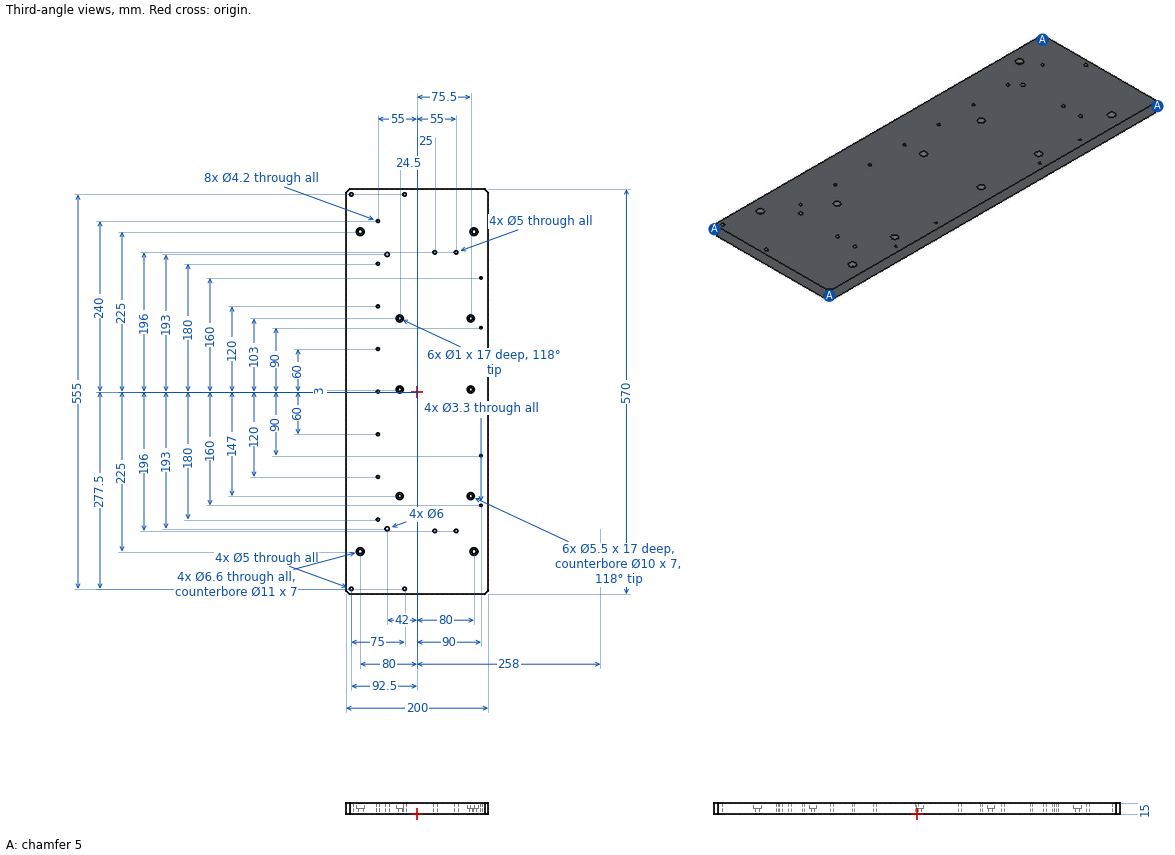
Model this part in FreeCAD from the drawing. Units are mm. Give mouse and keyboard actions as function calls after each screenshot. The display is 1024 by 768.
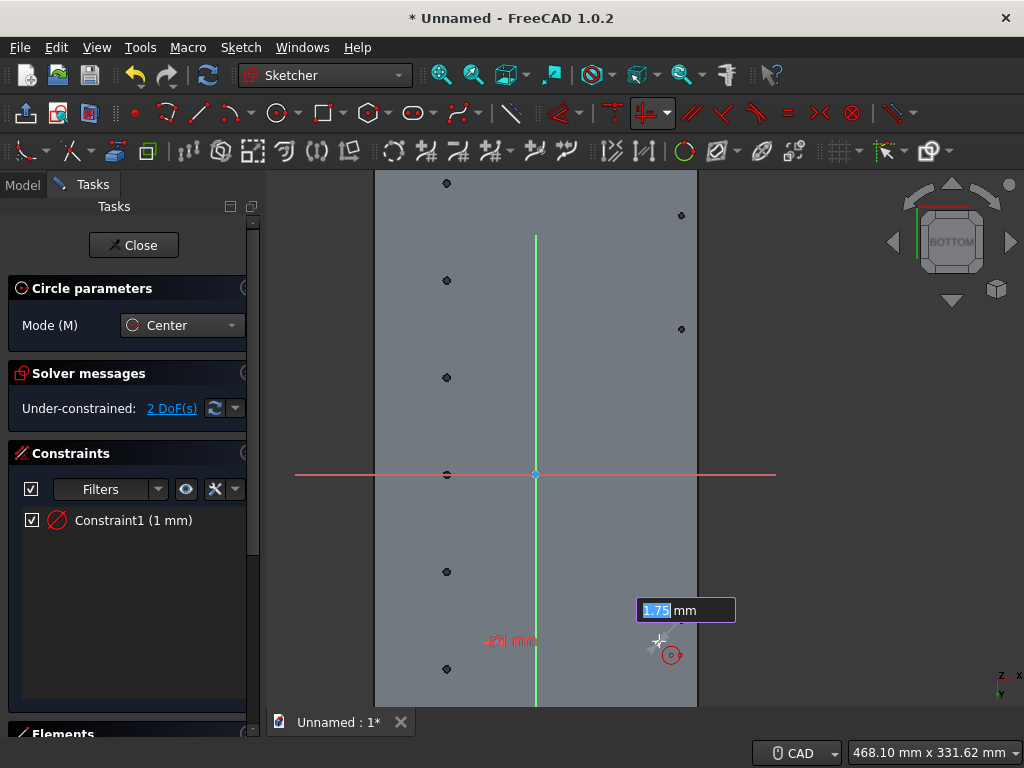
text(1)
key(Return)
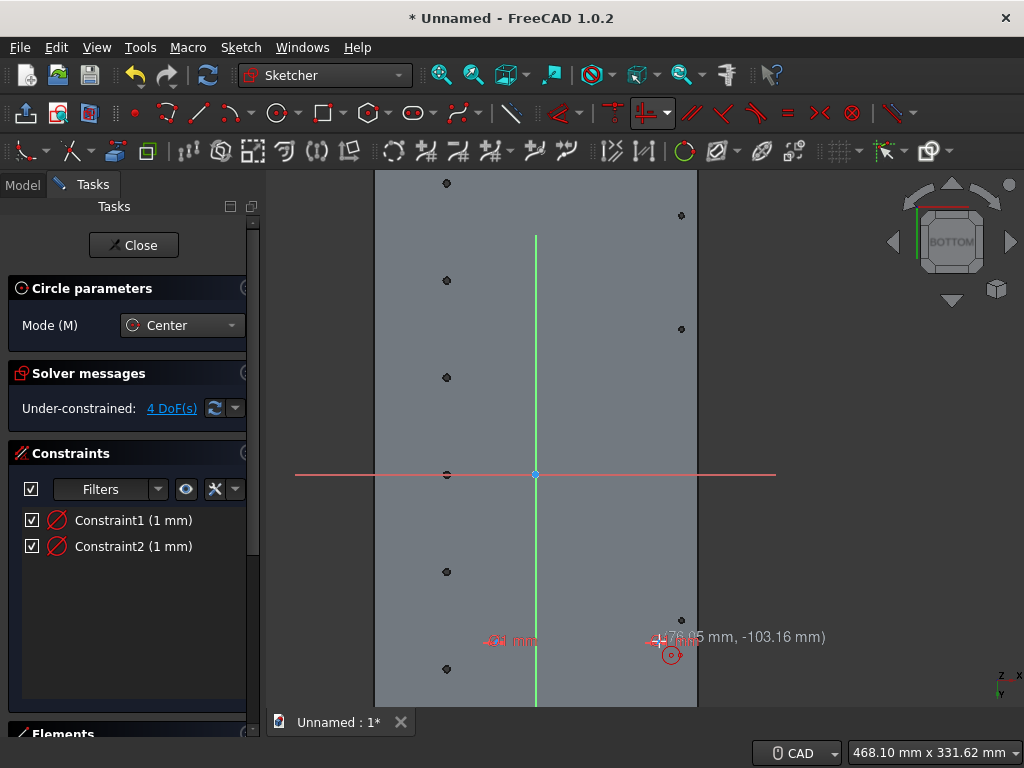
scroll(496, 237, up, 17)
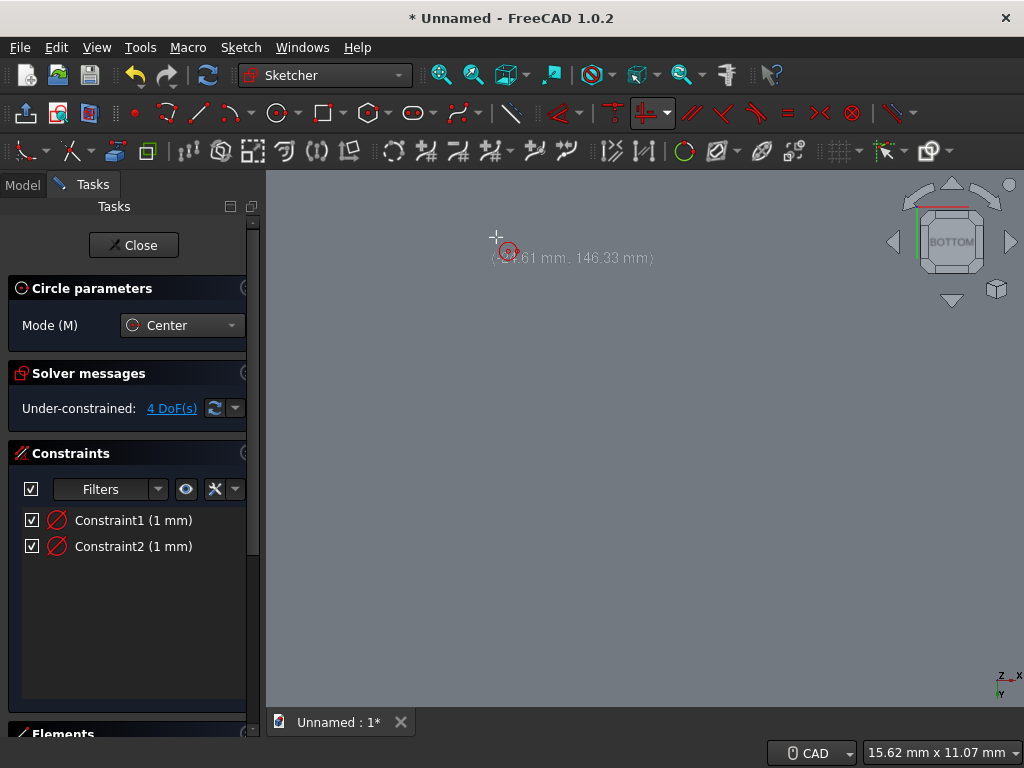
scroll(496, 236, down, 17)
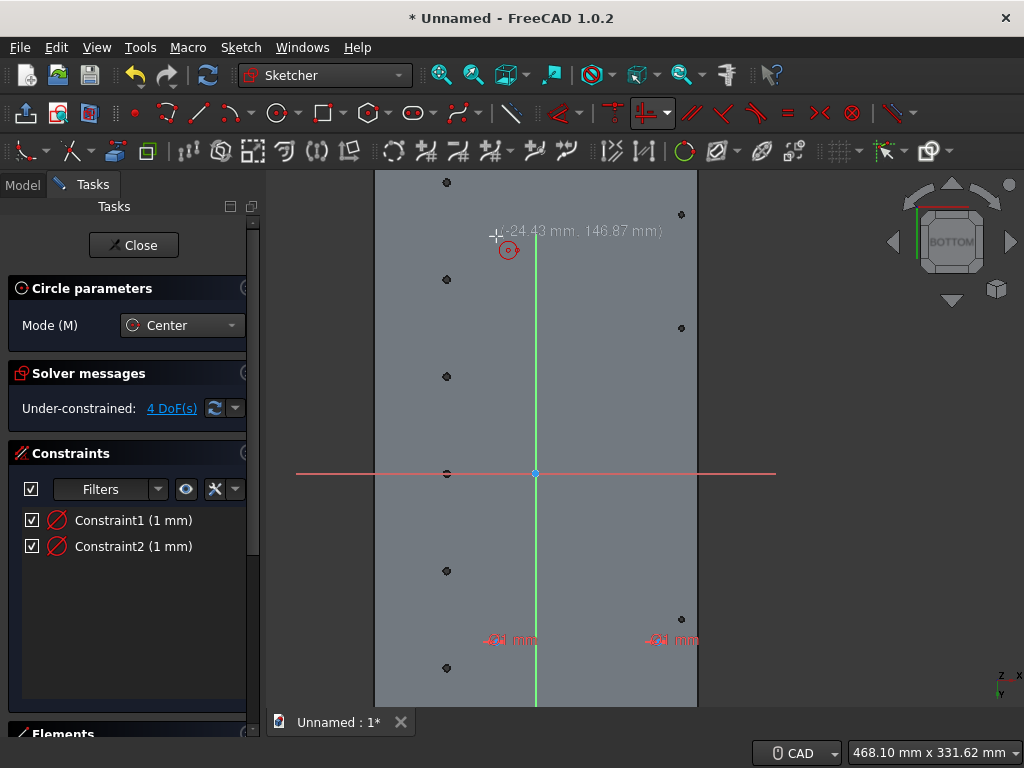
click(496, 236)
move(497, 235)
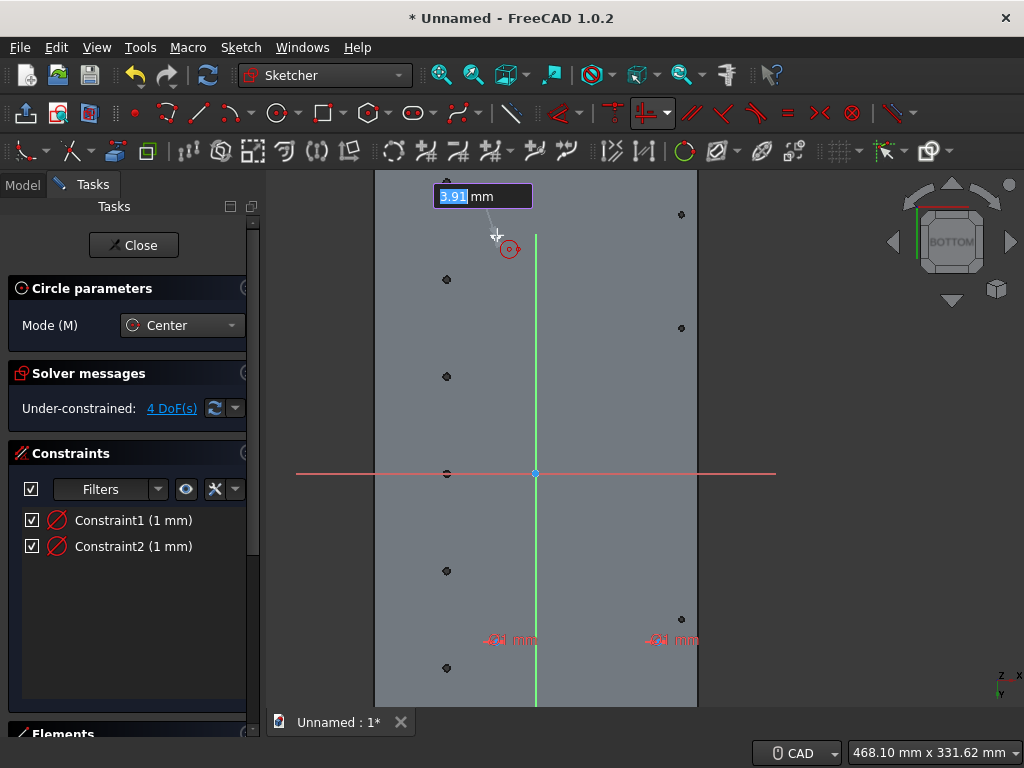
text(1)
key(Return)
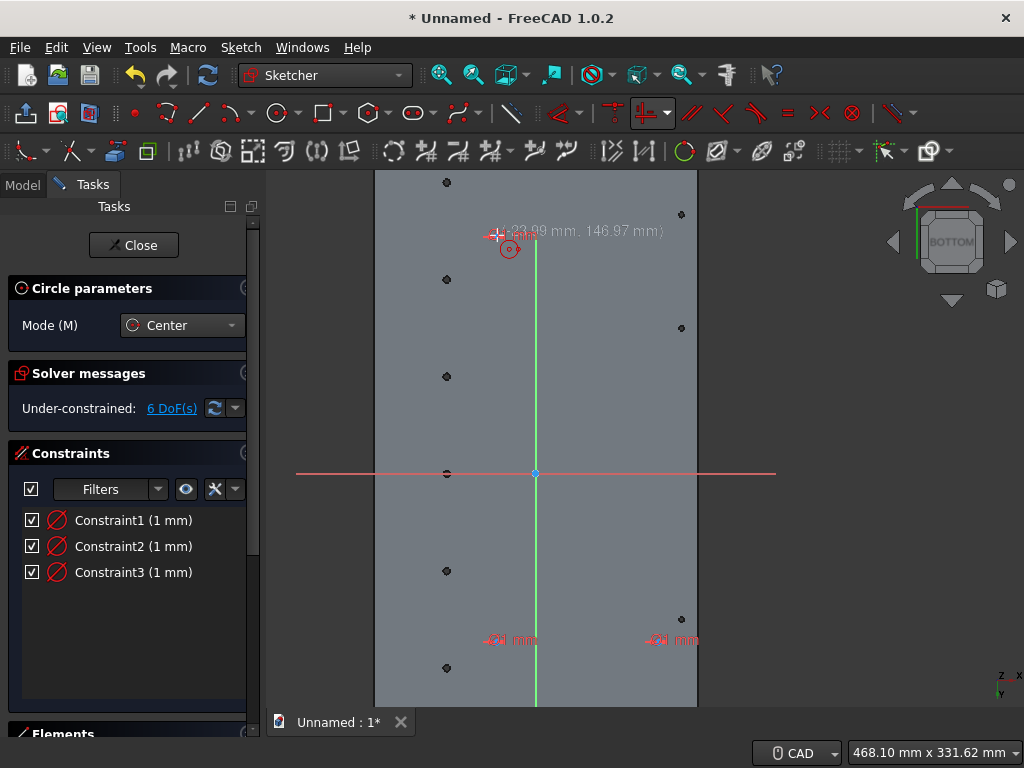
scroll(658, 236, up, 17)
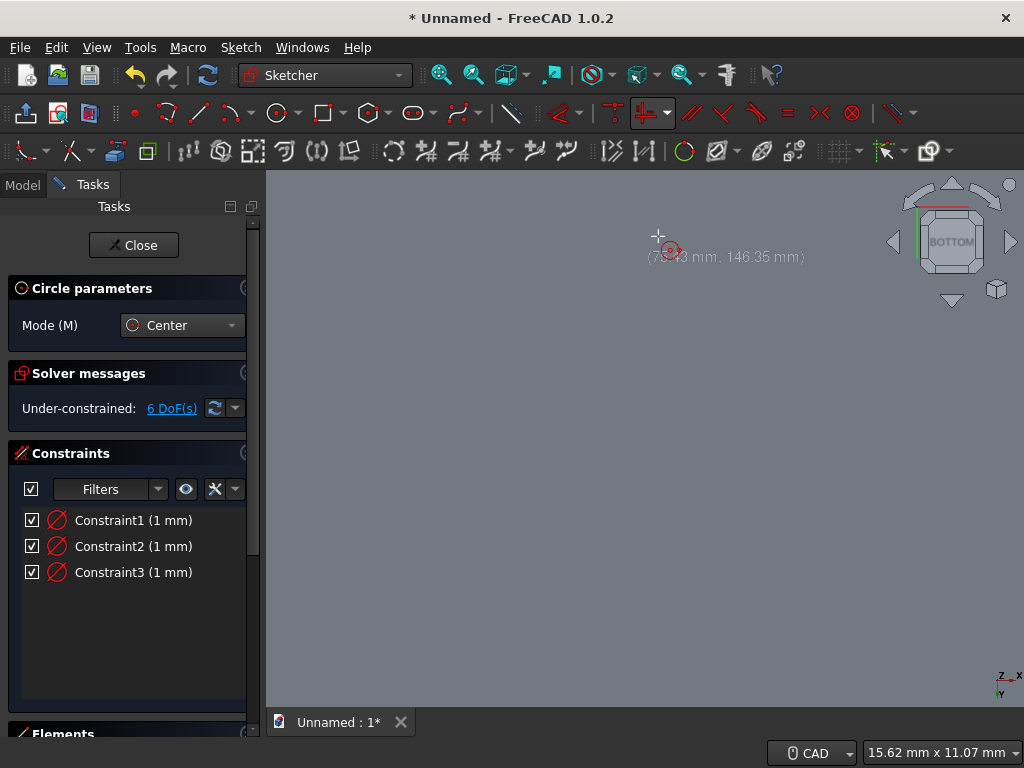
scroll(658, 236, down, 17)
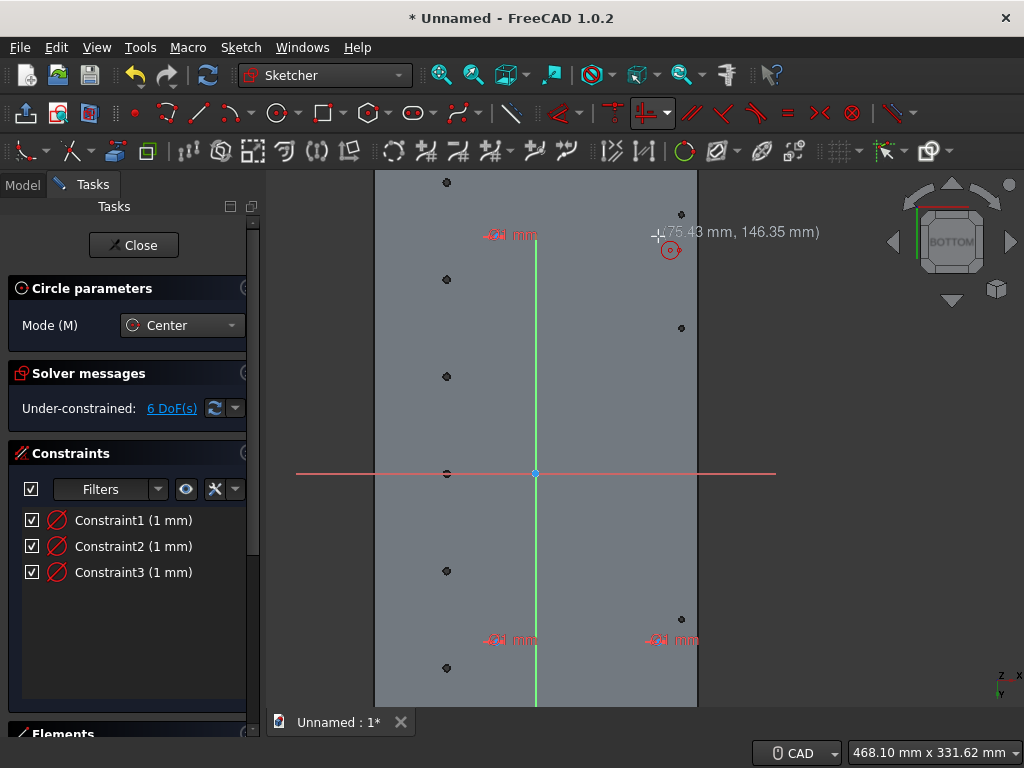
click(658, 236)
move(659, 235)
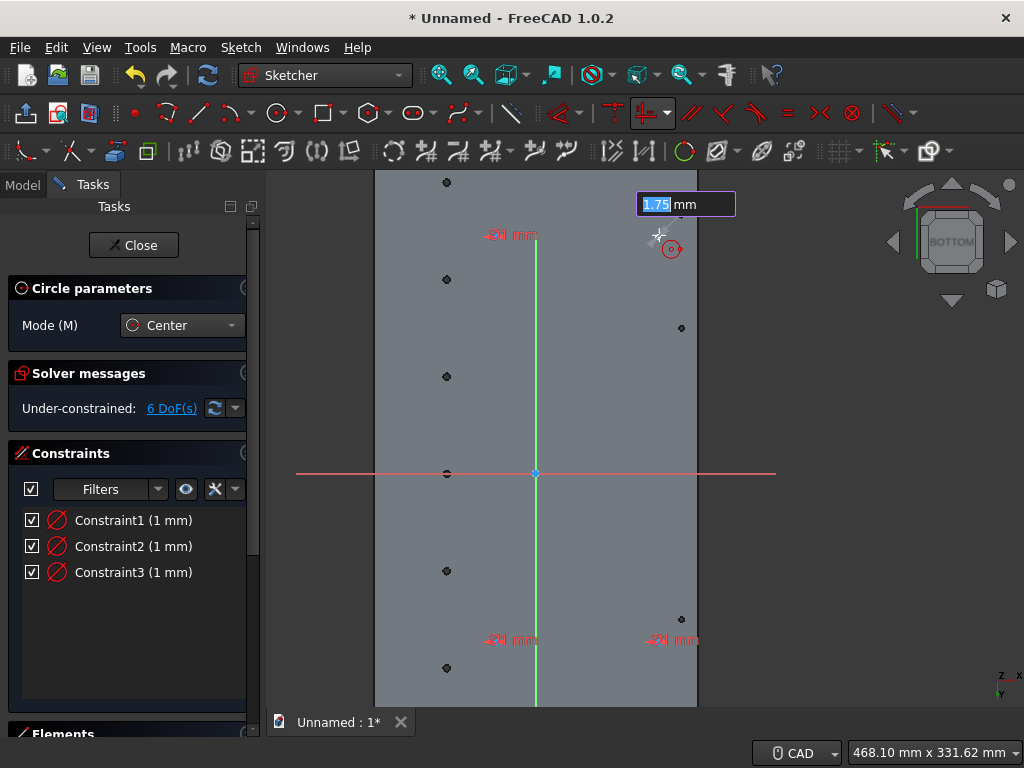
text(1)
key(Return)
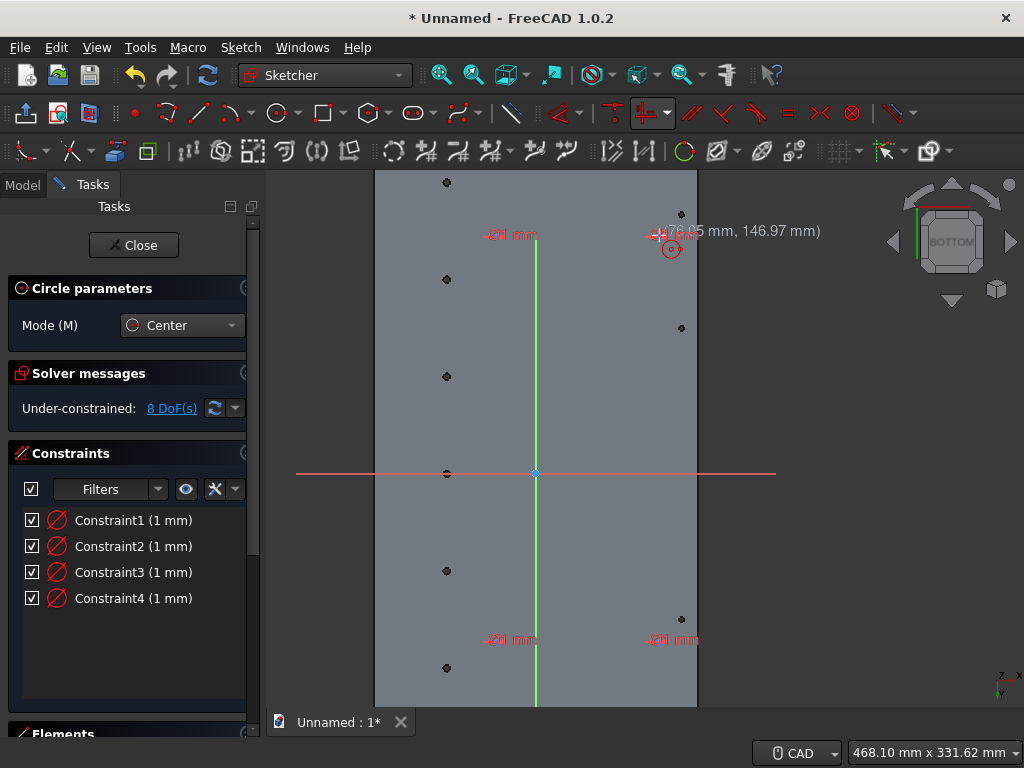
scroll(496, 479, up, 17)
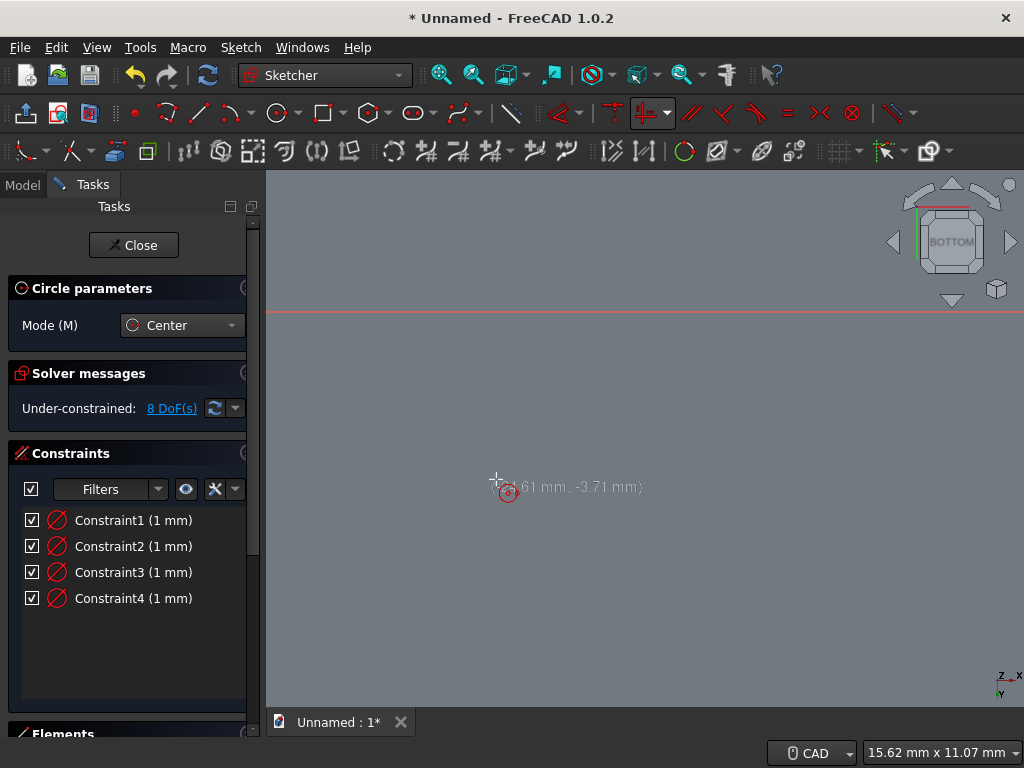
scroll(496, 480, down, 17)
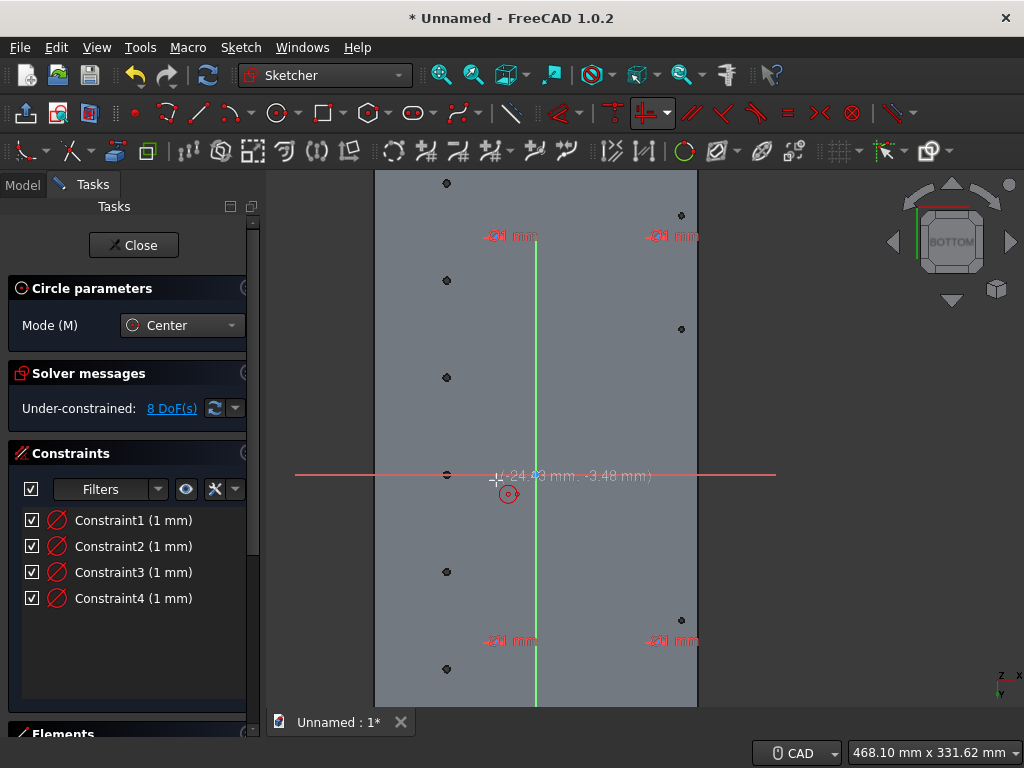
scroll(496, 480, up, 6)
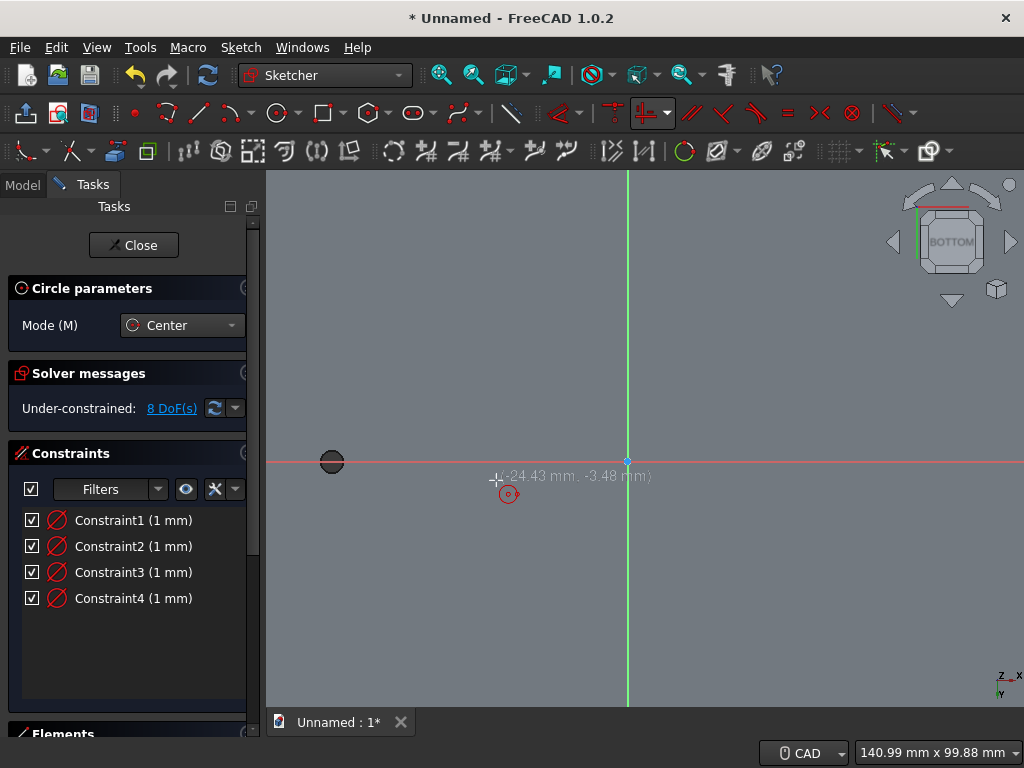
click(496, 478)
move(498, 476)